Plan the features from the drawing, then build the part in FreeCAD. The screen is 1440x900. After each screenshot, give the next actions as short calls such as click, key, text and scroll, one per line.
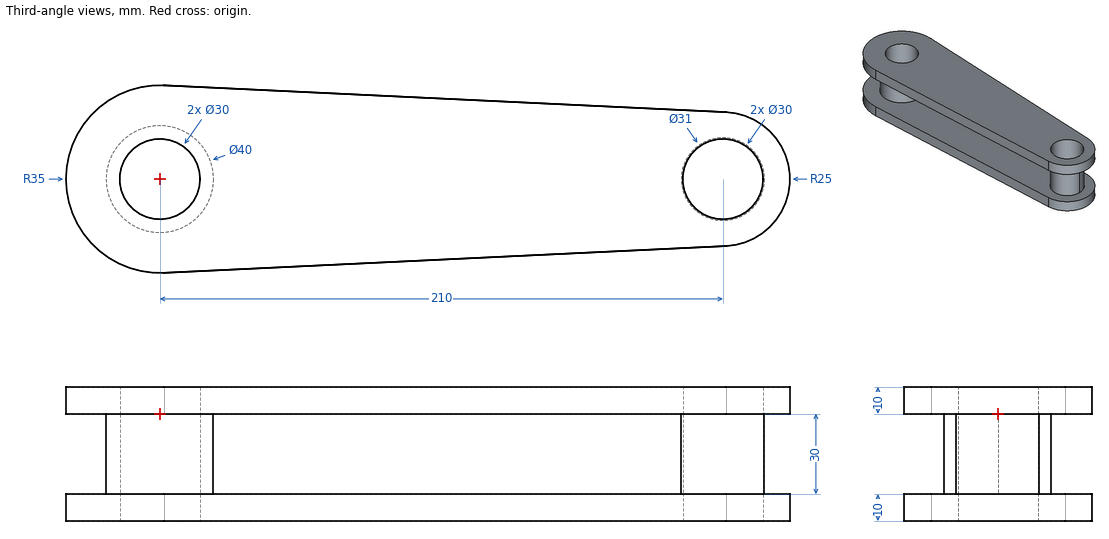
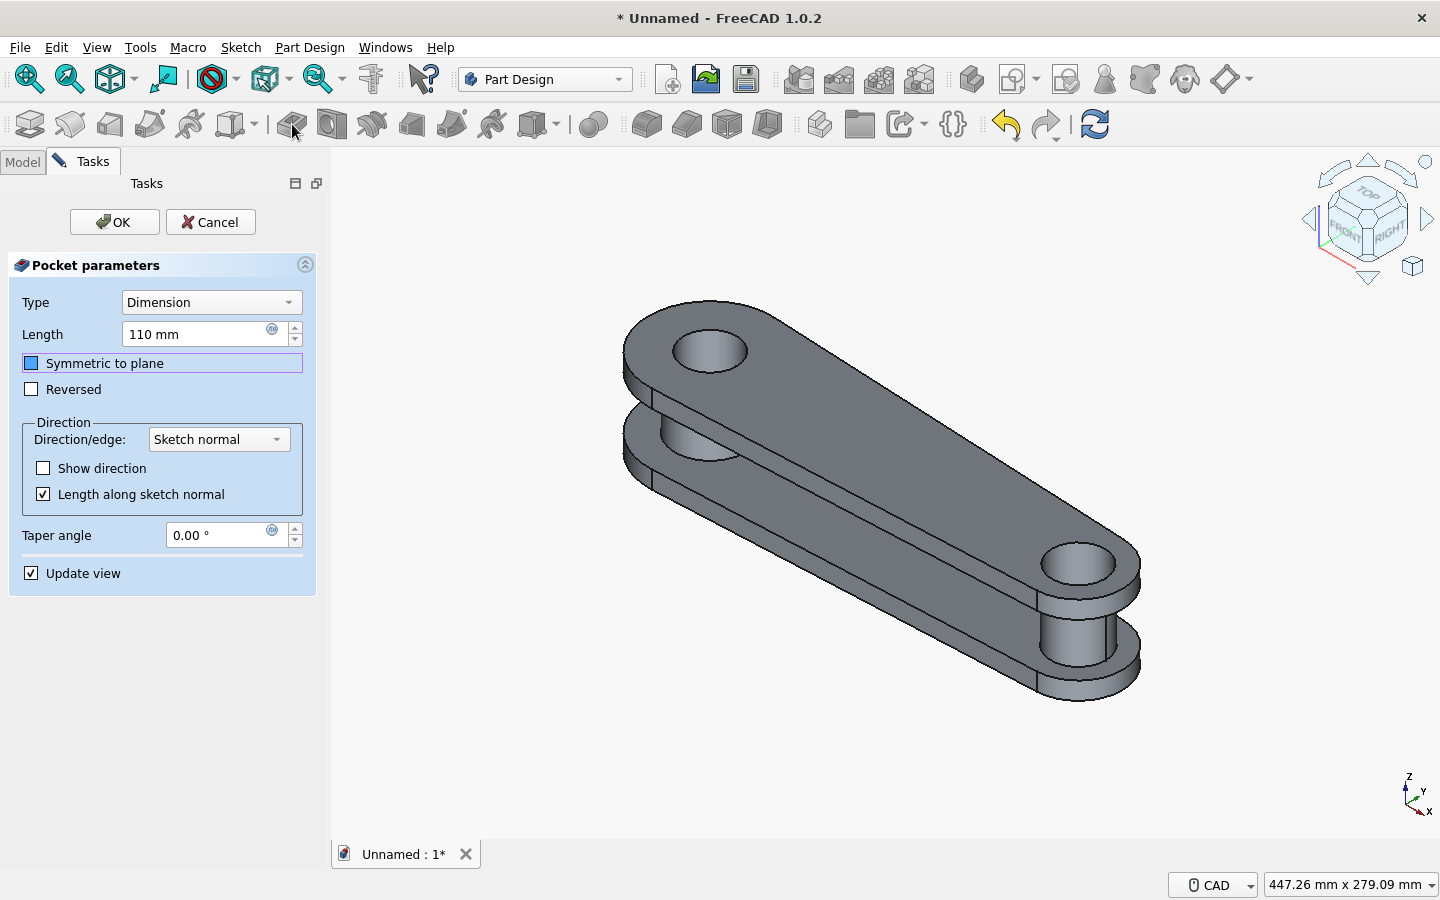
click(115, 222)